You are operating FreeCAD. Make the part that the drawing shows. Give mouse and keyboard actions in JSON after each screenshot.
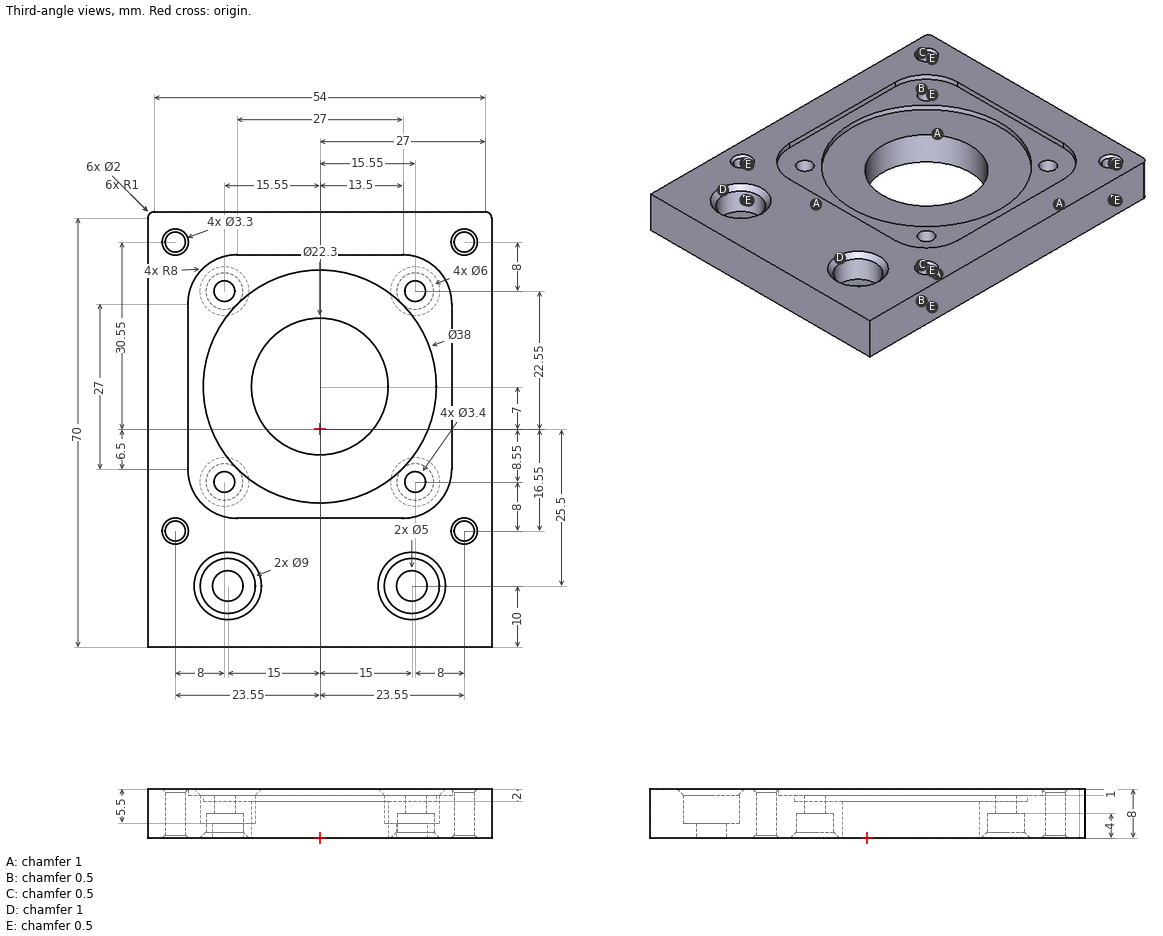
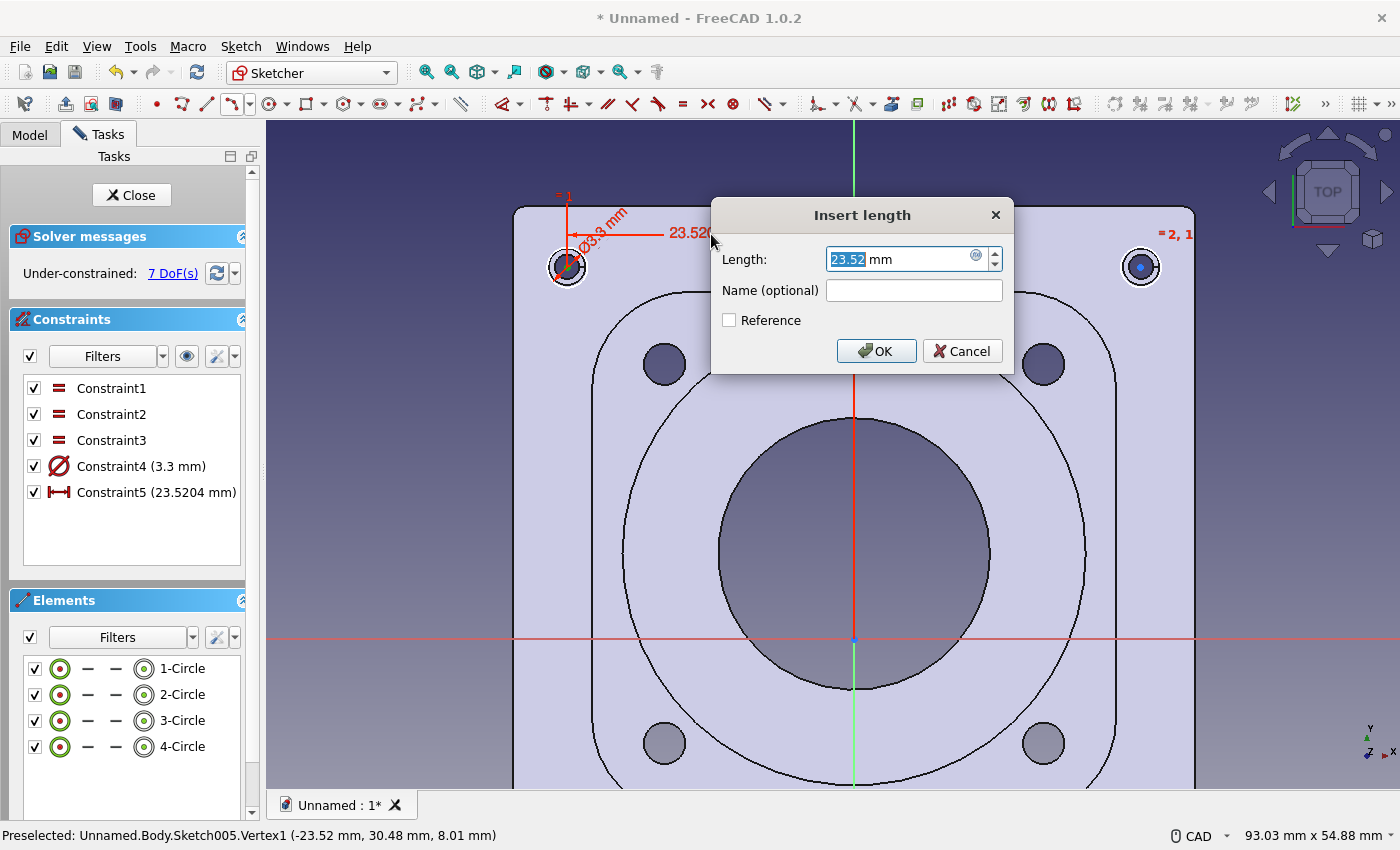
{"action": "type", "text": "23.55"}
{"action": "key", "text": "Return"}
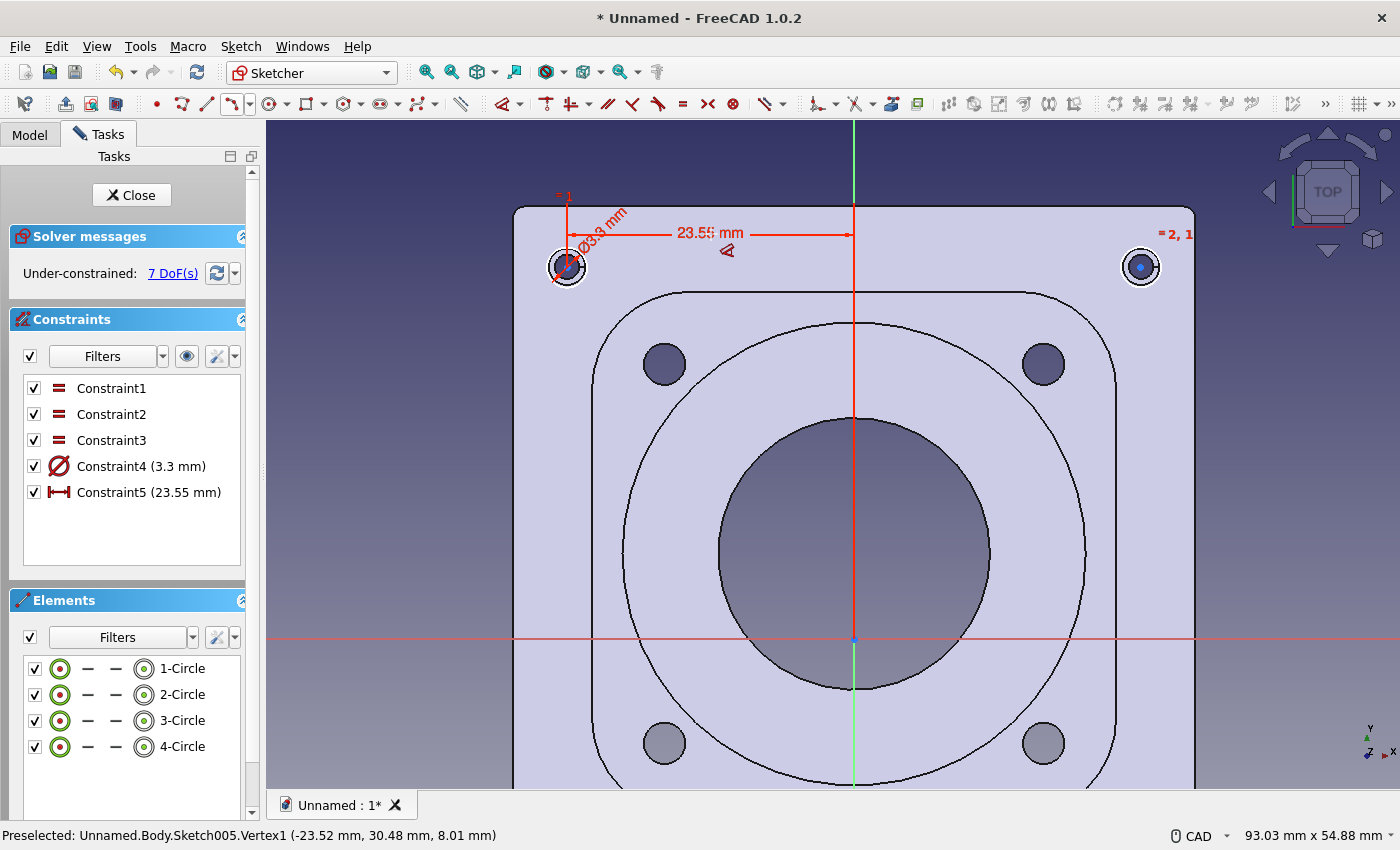
{"action": "left_click", "coordinate": [567, 268]}
{"action": "left_click", "coordinate": [533, 453]}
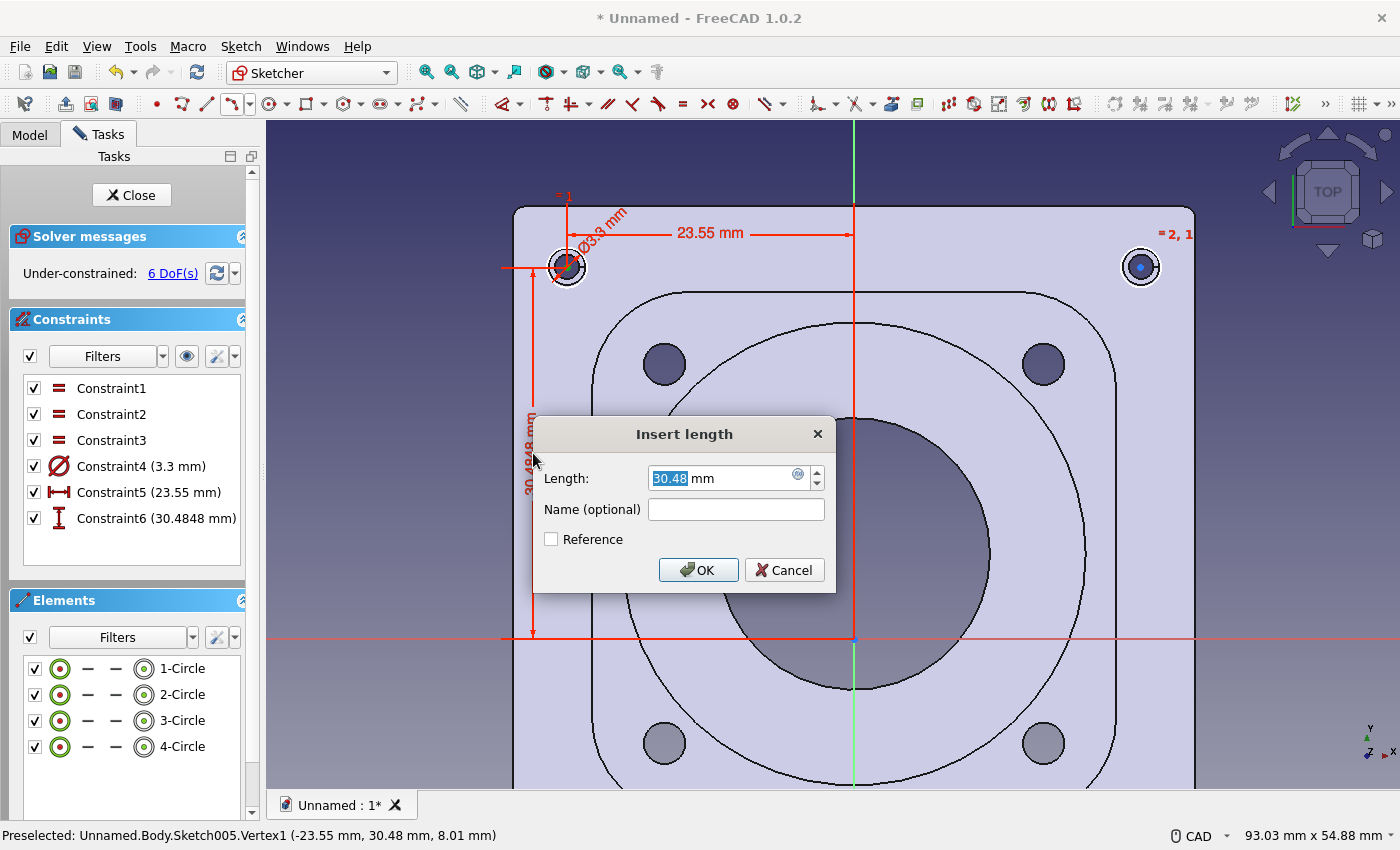
{"action": "type", "text": "30.55"}
{"action": "key", "text": "Return"}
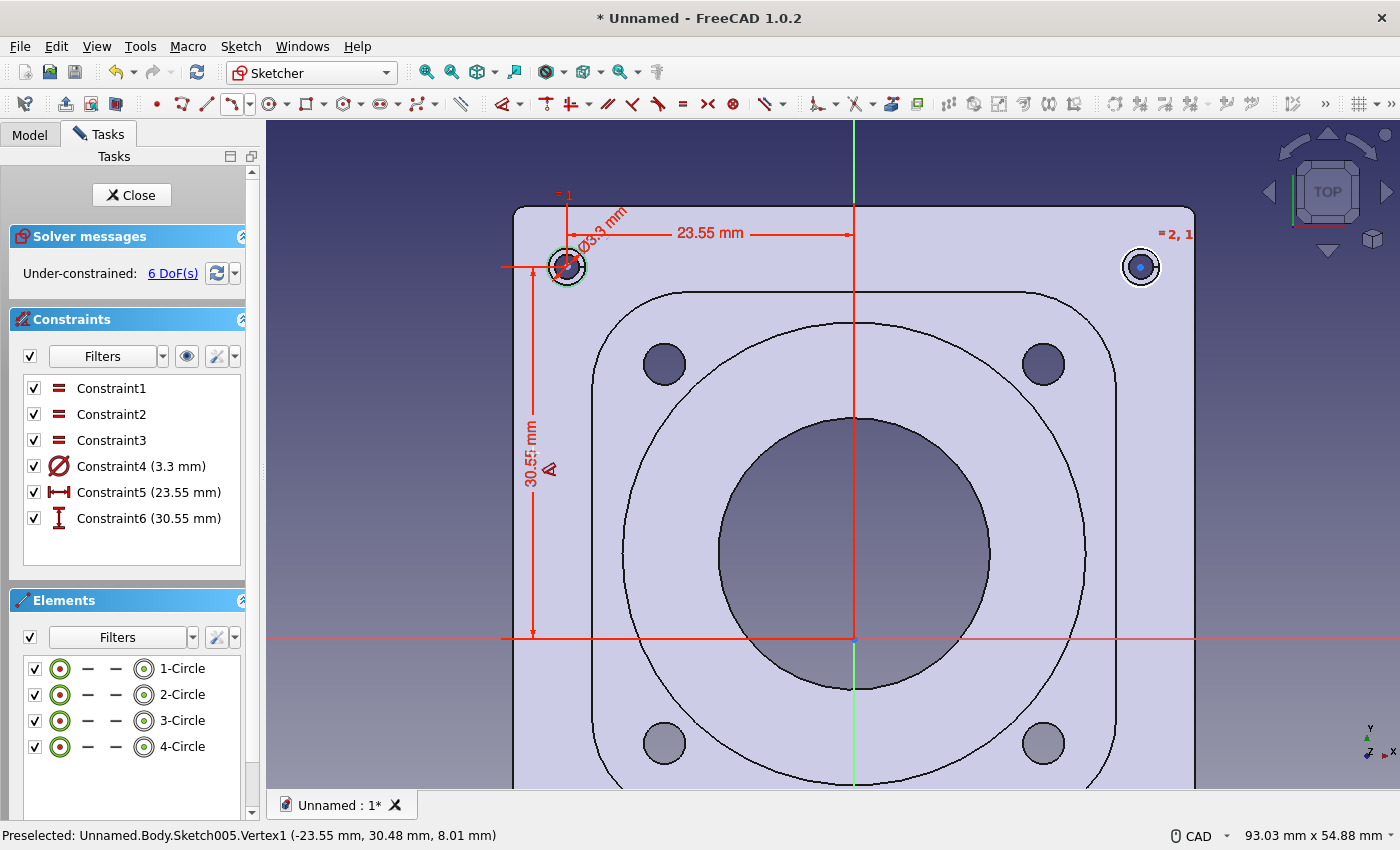
{"action": "left_click", "coordinate": [1141, 267]}
{"action": "left_click", "coordinate": [997, 233]}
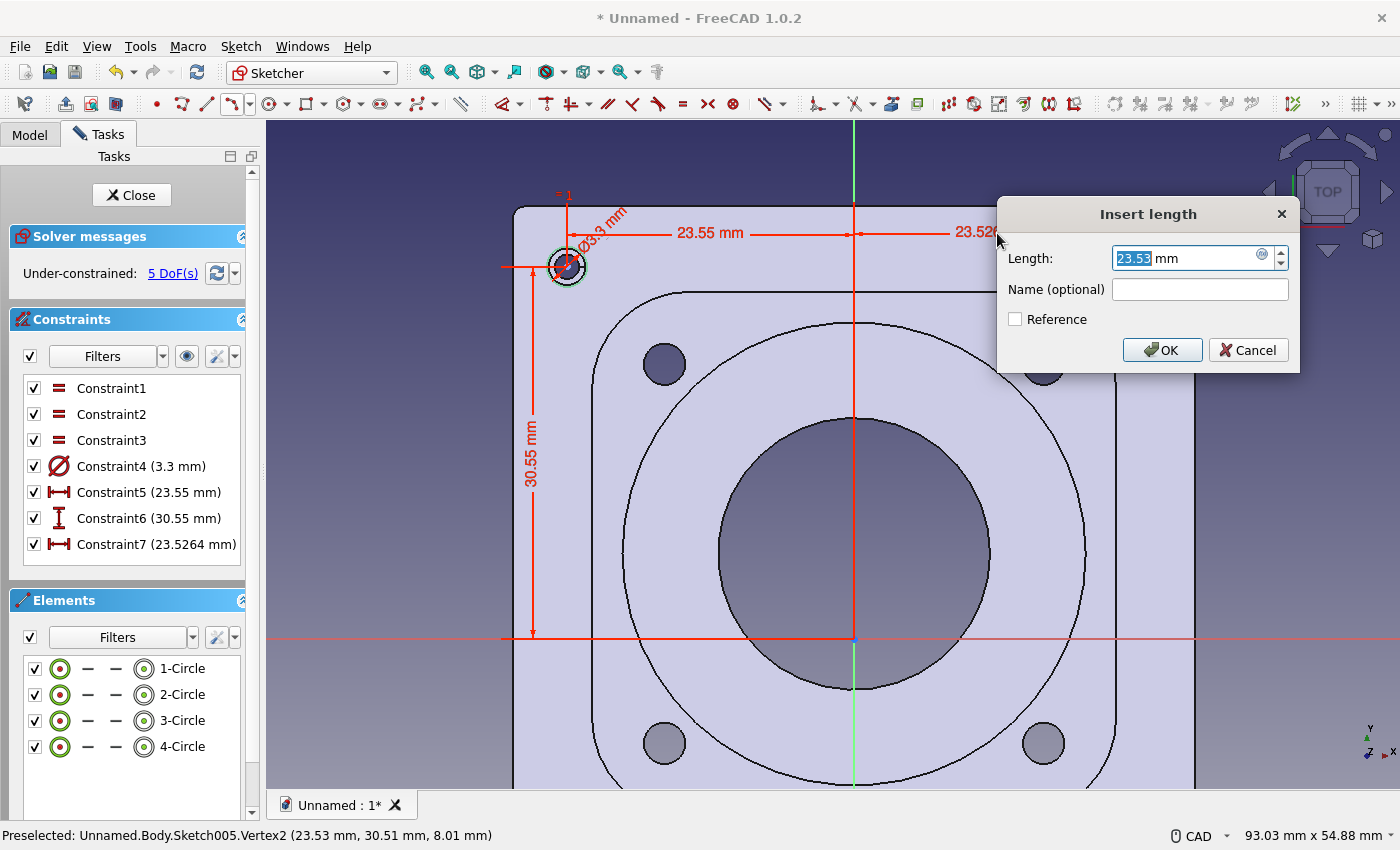
{"action": "type", "text": "23.55"}
{"action": "key", "text": "Return"}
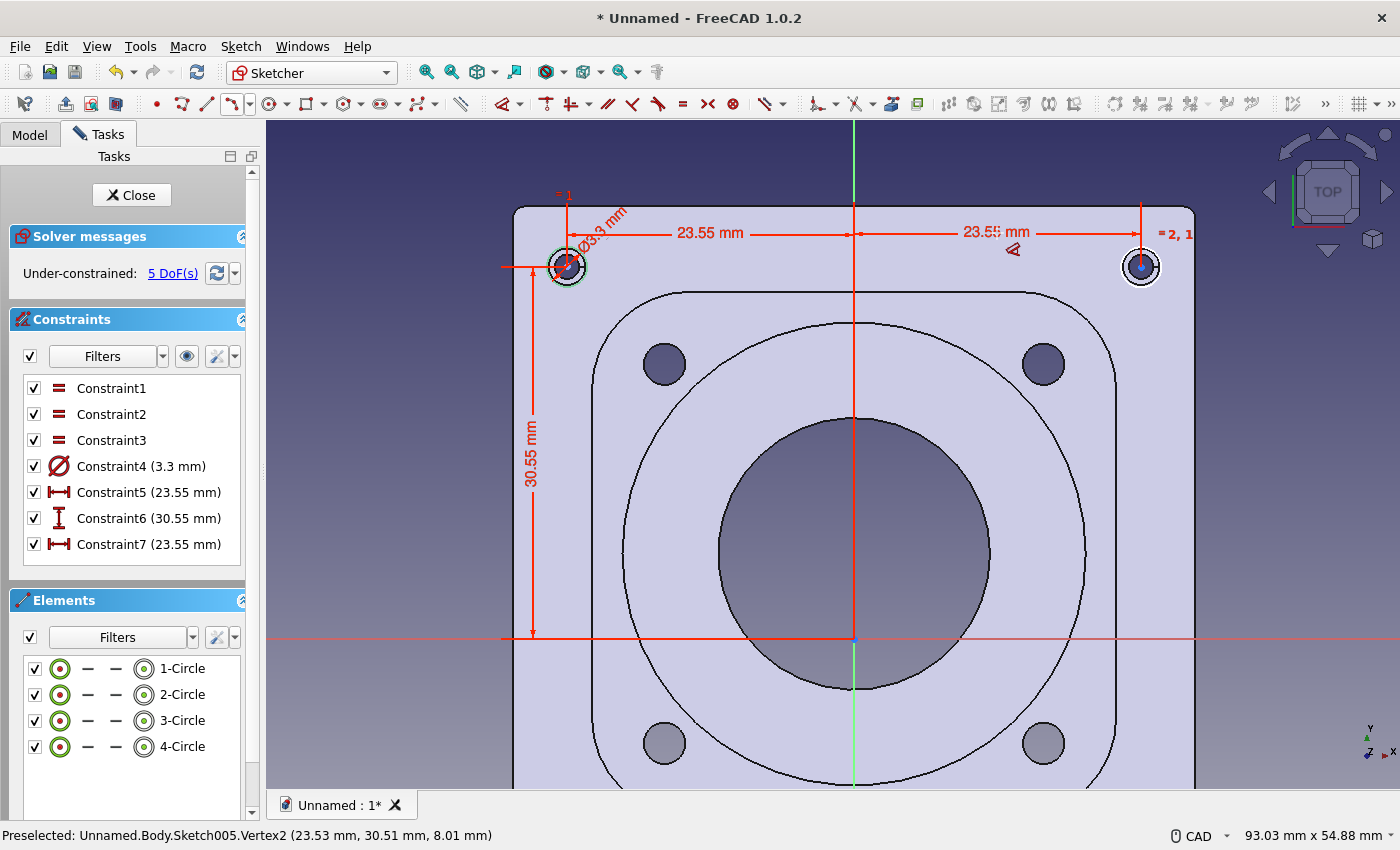
{"action": "left_click", "coordinate": [1141, 267]}
{"action": "left_click", "coordinate": [1175, 453]}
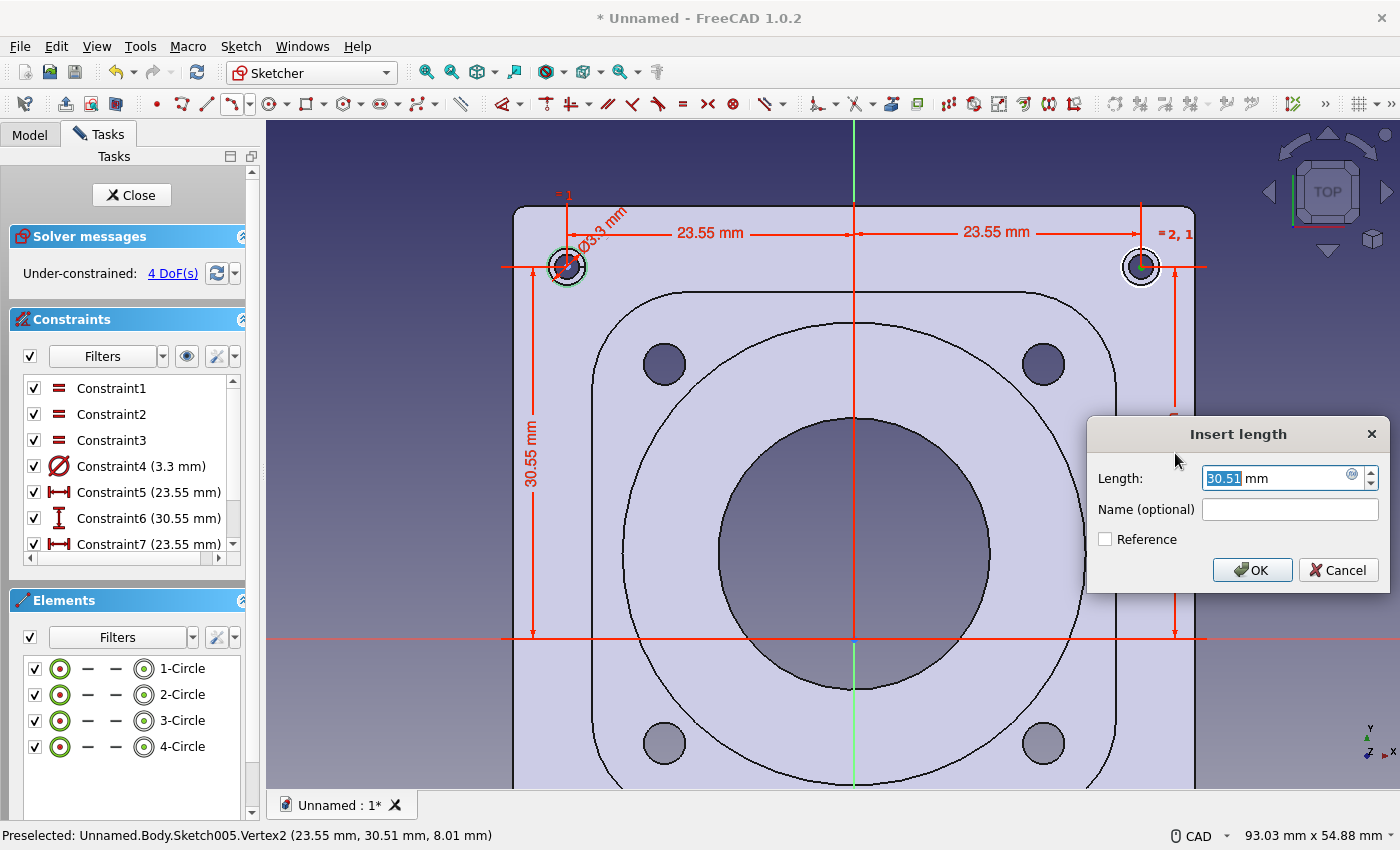
{"action": "type", "text": "30.55"}
{"action": "key", "text": "Return"}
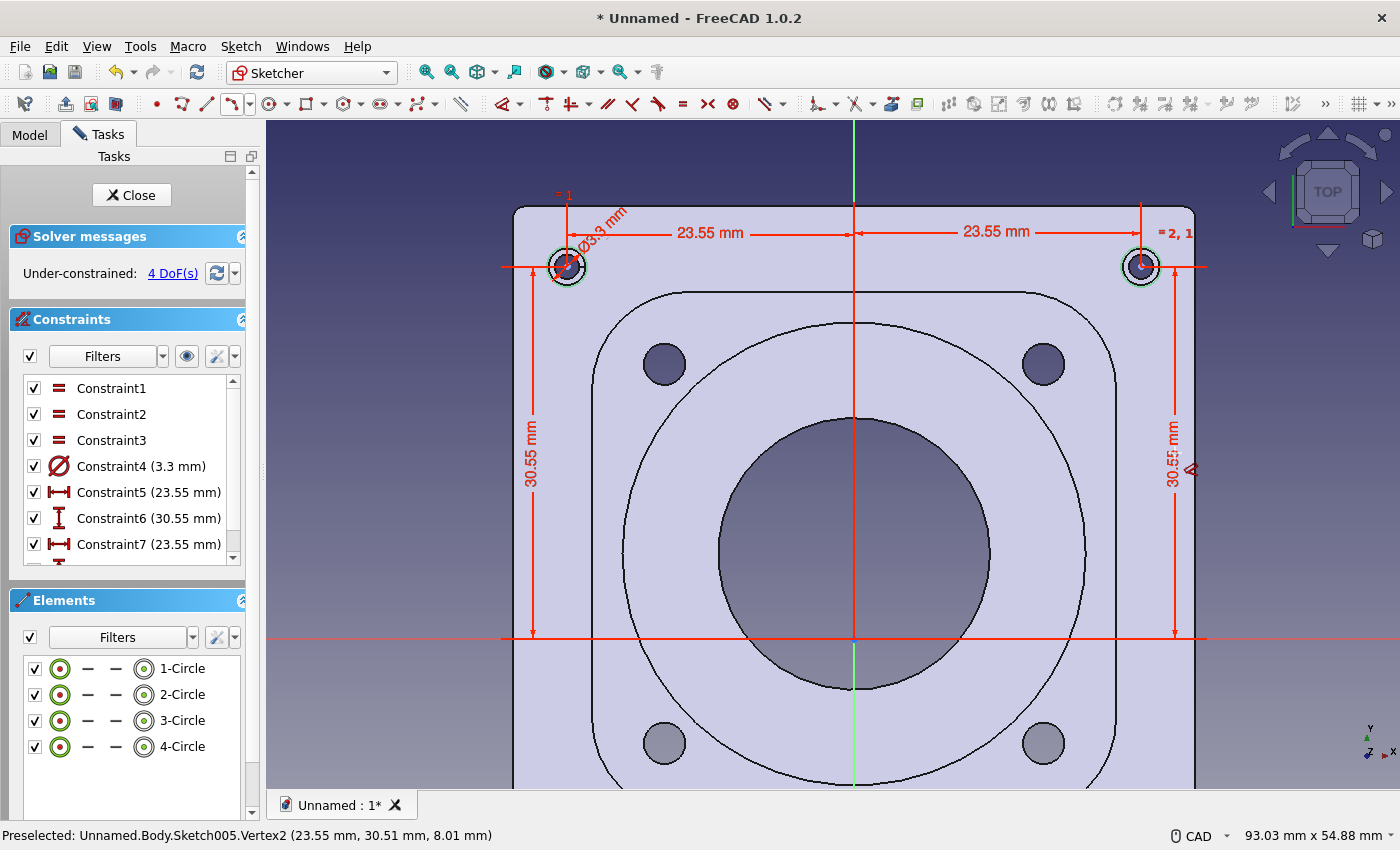
{"action": "scroll", "coordinate": [582, 252], "scroll_direction": "down", "scroll_amount": 2}